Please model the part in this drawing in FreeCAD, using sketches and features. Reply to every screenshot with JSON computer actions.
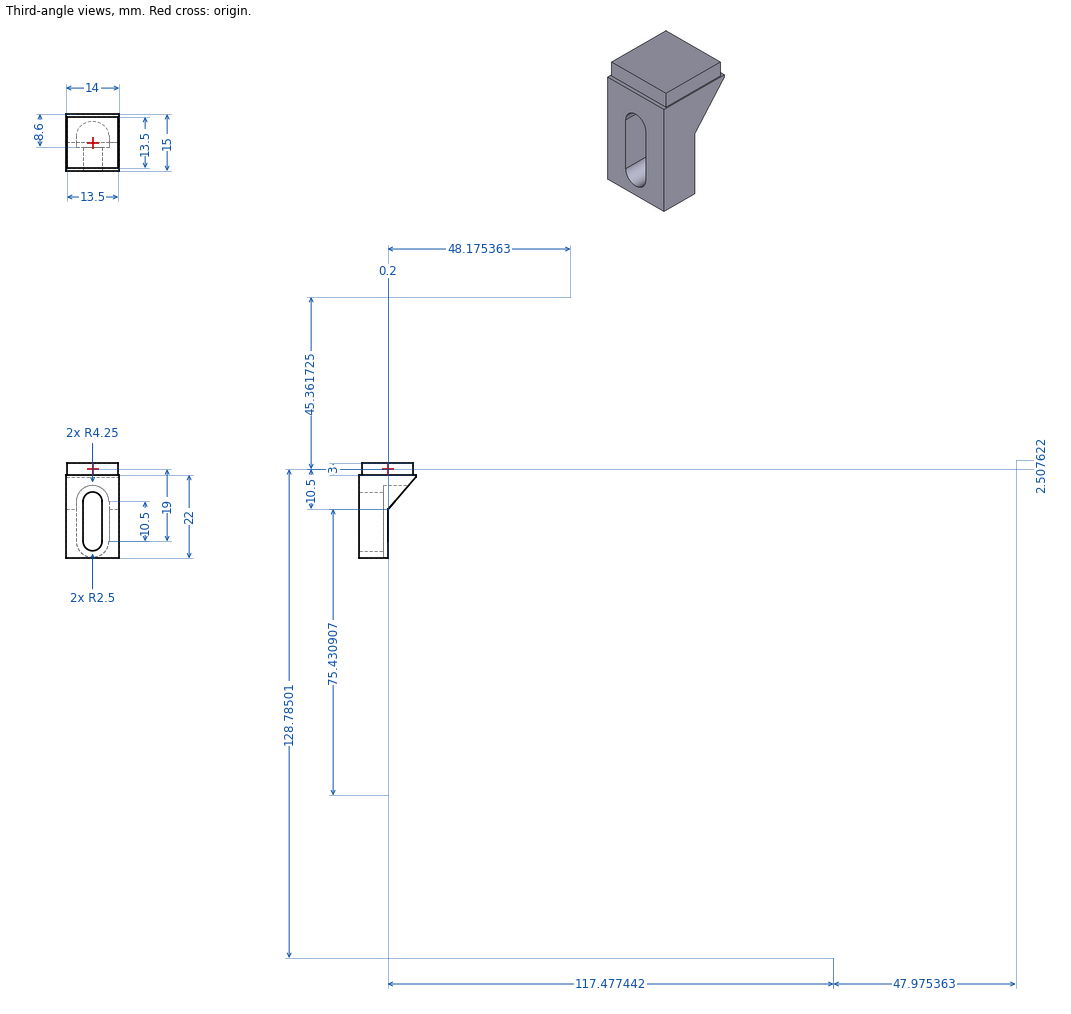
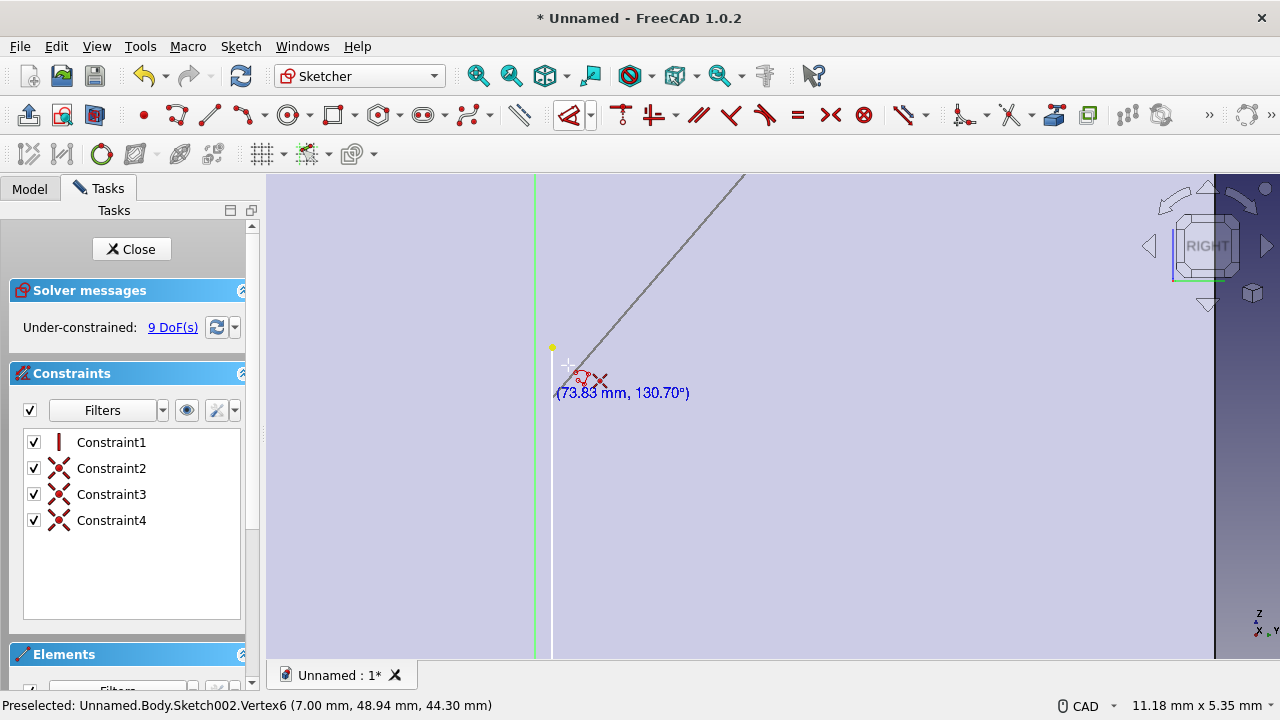
{"action": "left_click", "coordinate": [552, 348]}
{"action": "key", "text": "Escape"}
{"action": "key", "text": "Escape"}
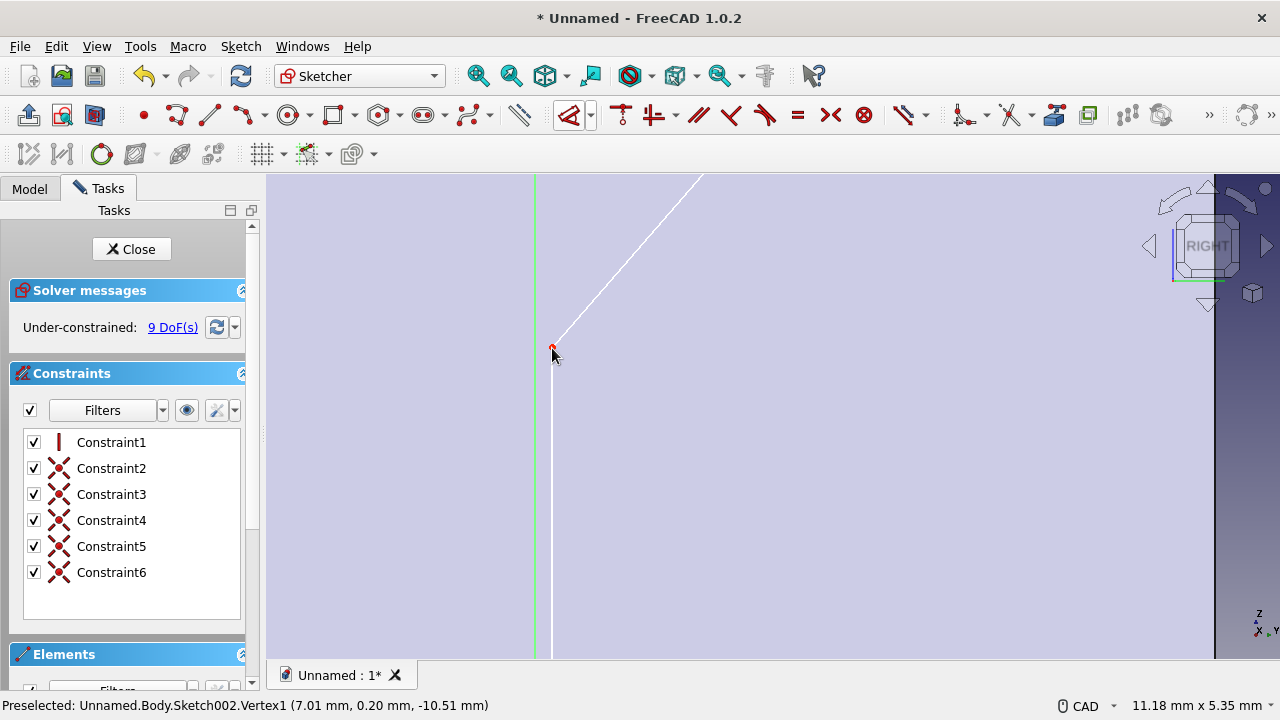
{"action": "scroll", "coordinate": [552, 348], "scroll_direction": "up", "scroll_amount": 4}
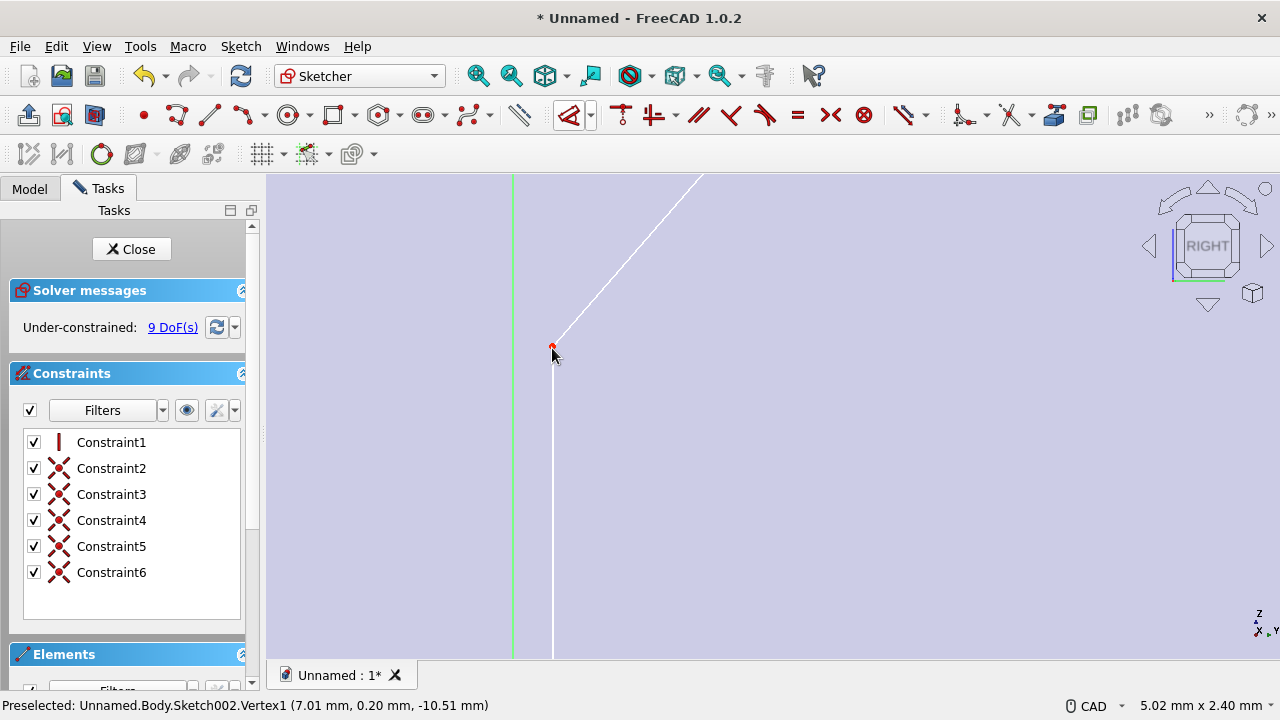
{"action": "left_click", "coordinate": [553, 347]}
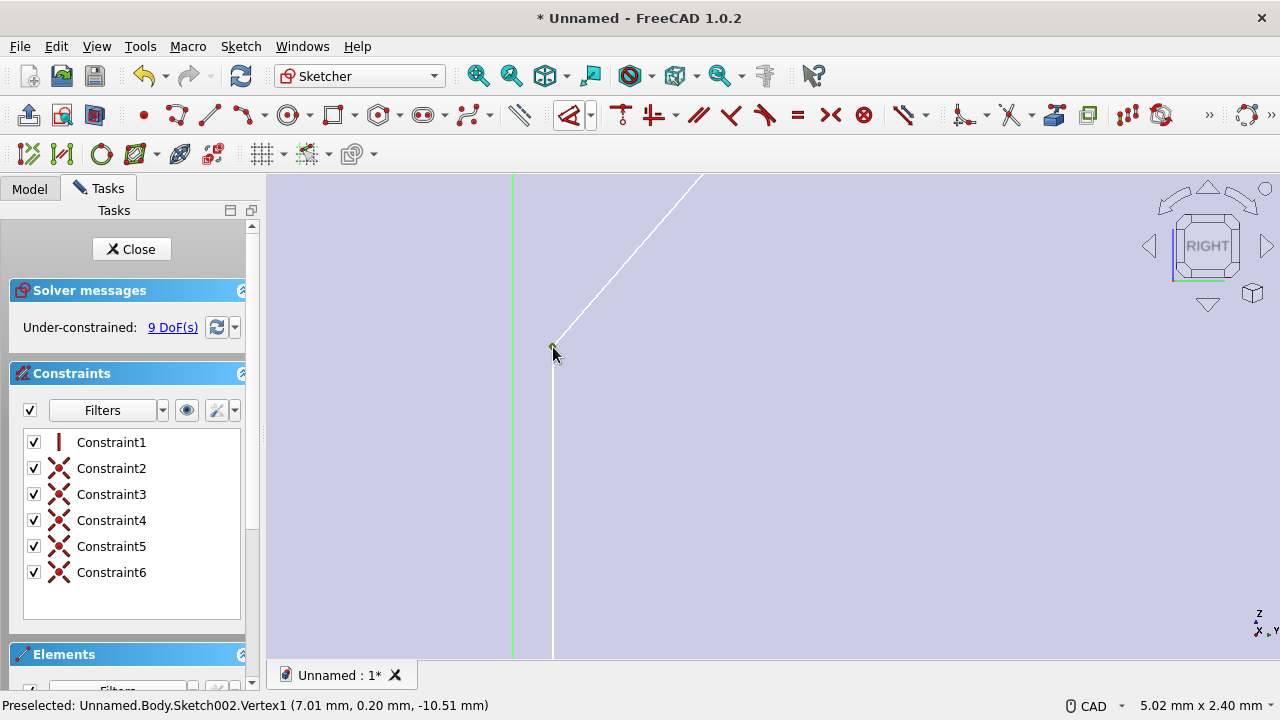
{"action": "key", "text": "l"}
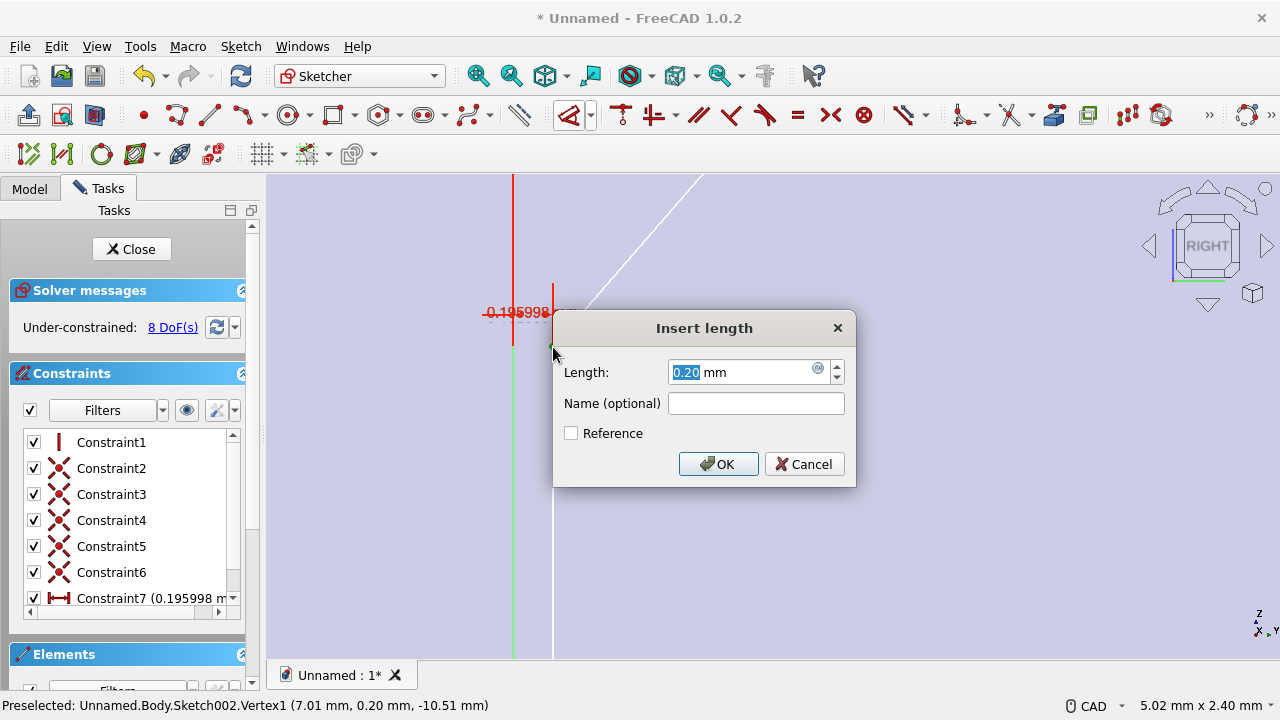
{"action": "type", "text": "0.2"}
{"action": "key", "text": "Return"}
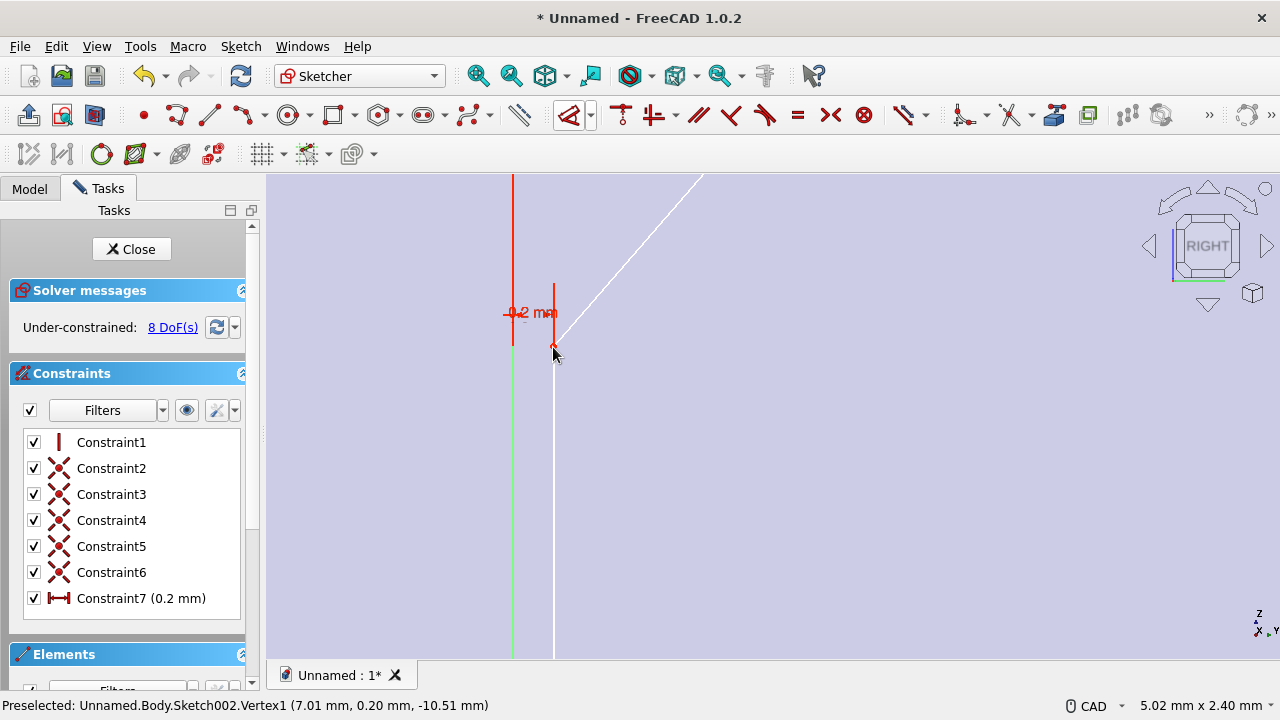
{"action": "scroll", "coordinate": [704, 416], "scroll_direction": "down", "scroll_amount": 15}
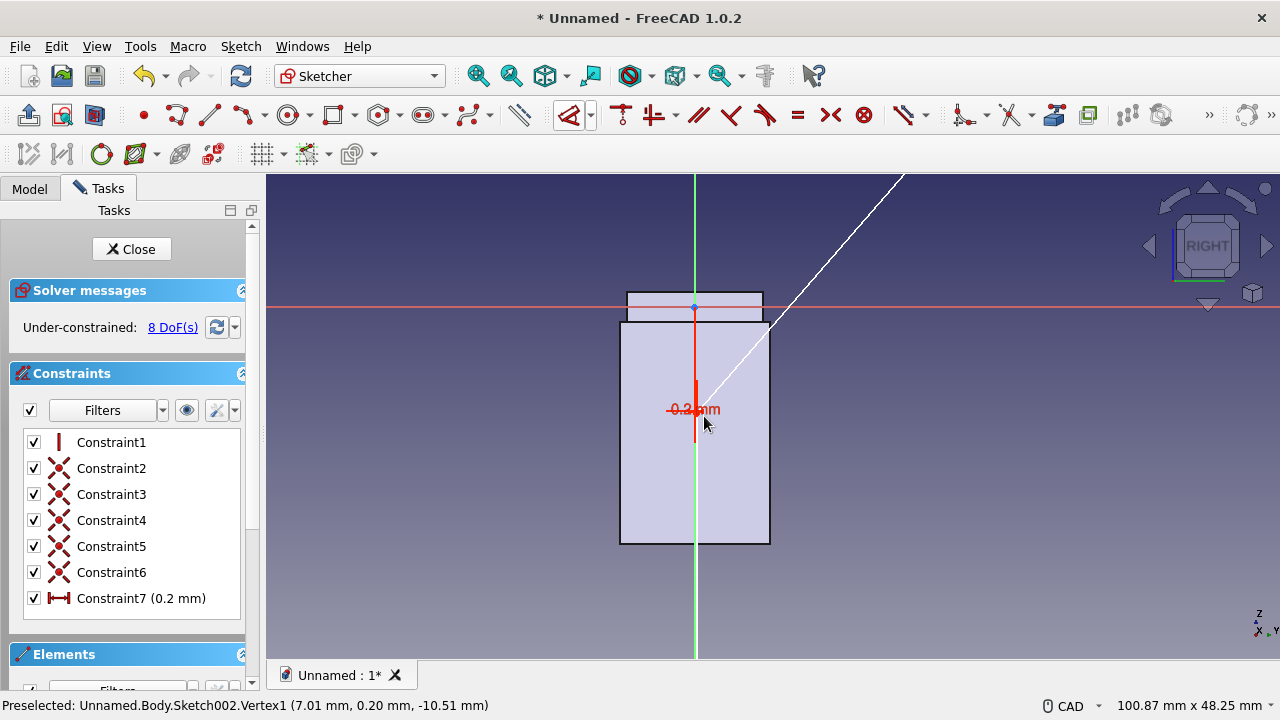
{"action": "scroll", "coordinate": [542, 355], "scroll_direction": "down", "scroll_amount": 9}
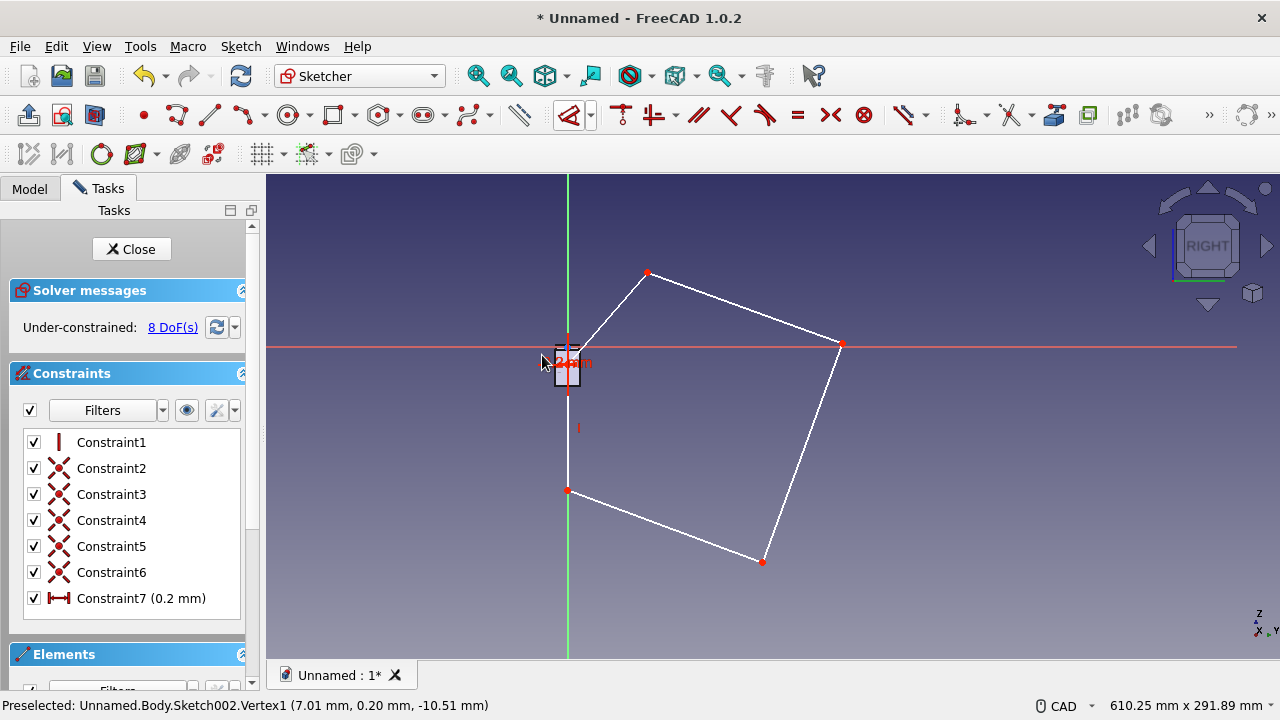
{"action": "scroll", "coordinate": [568, 365], "scroll_direction": "up", "scroll_amount": 5}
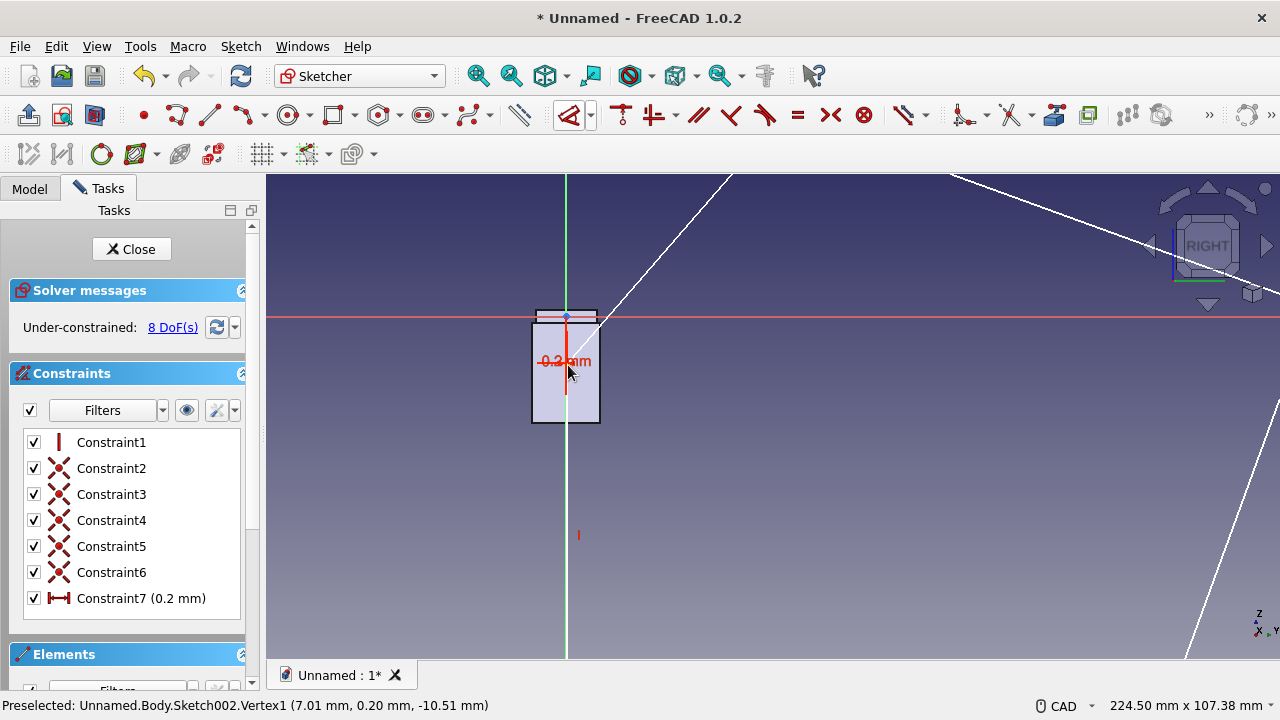
{"action": "left_click", "coordinate": [567, 364]}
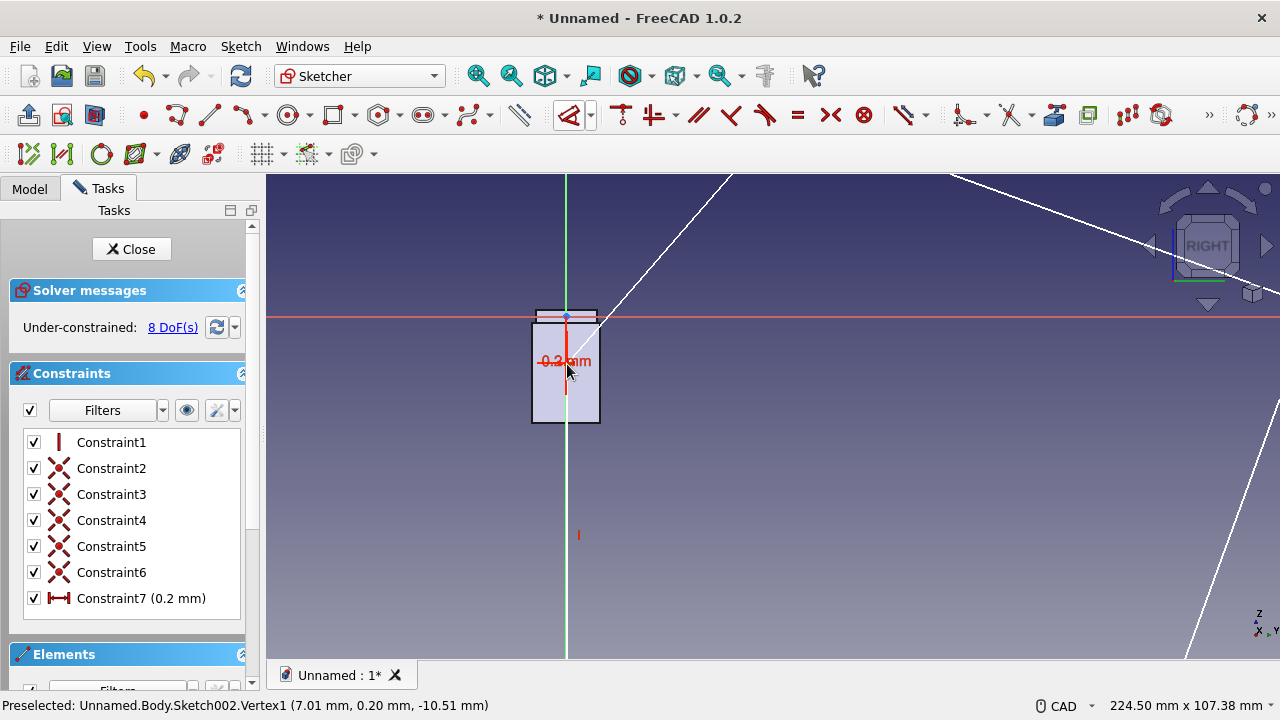
{"action": "key", "text": "i"}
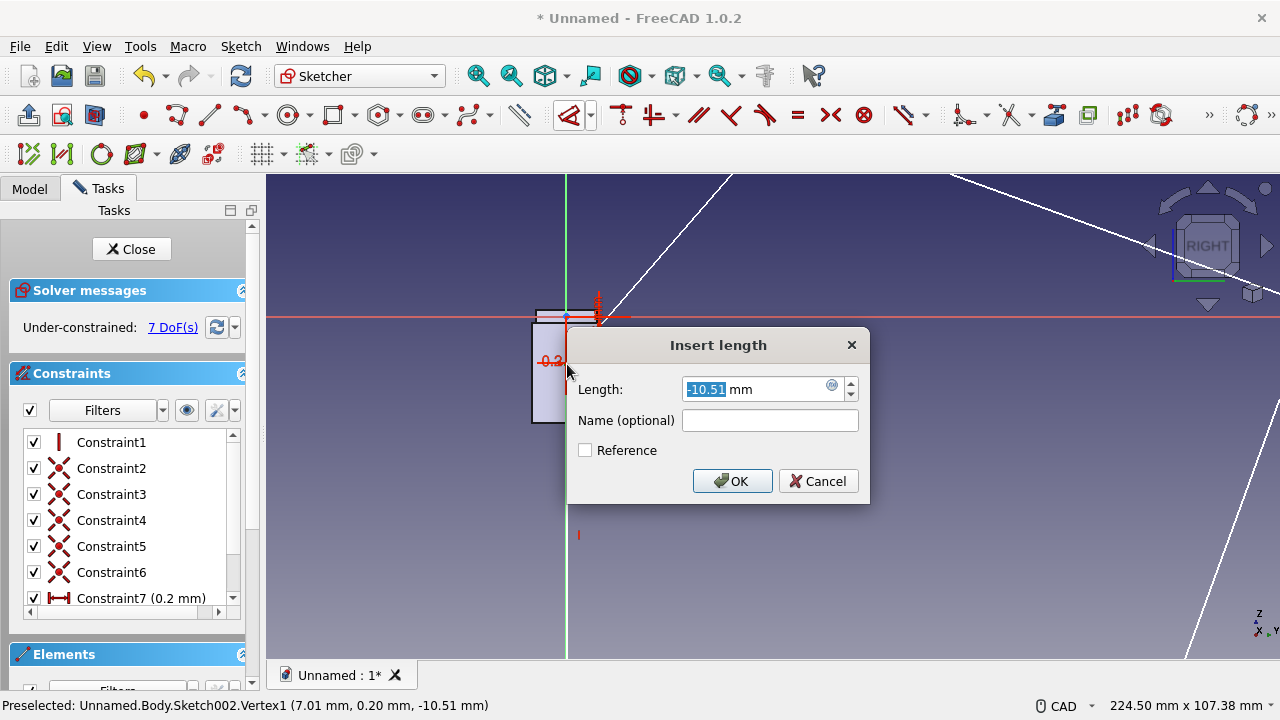
{"action": "type", "text": "-10.5"}
{"action": "key", "text": "Return"}